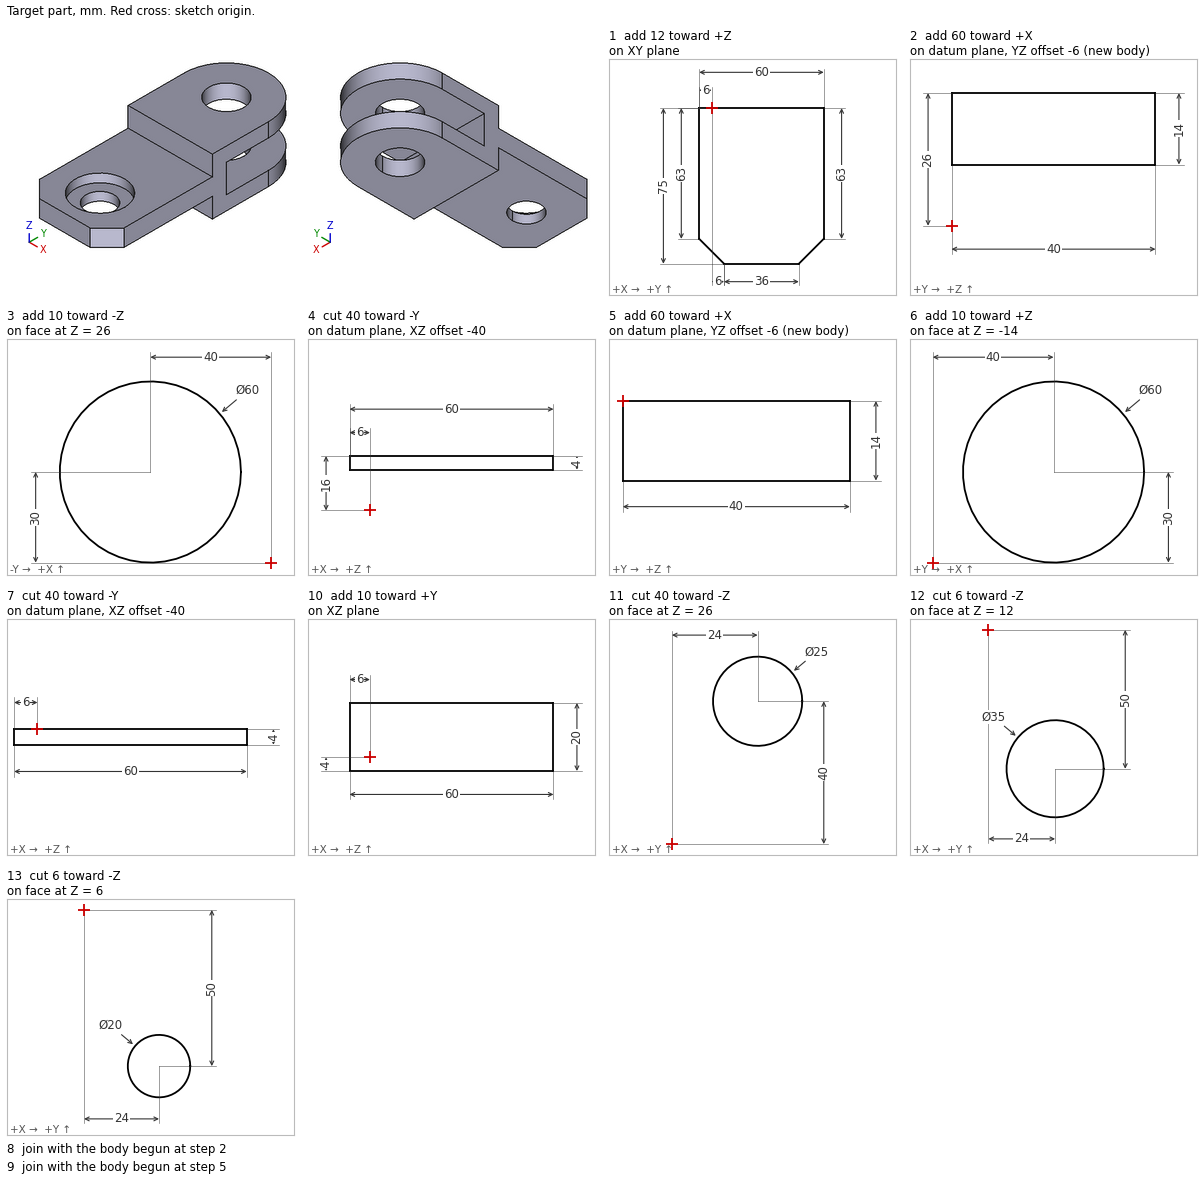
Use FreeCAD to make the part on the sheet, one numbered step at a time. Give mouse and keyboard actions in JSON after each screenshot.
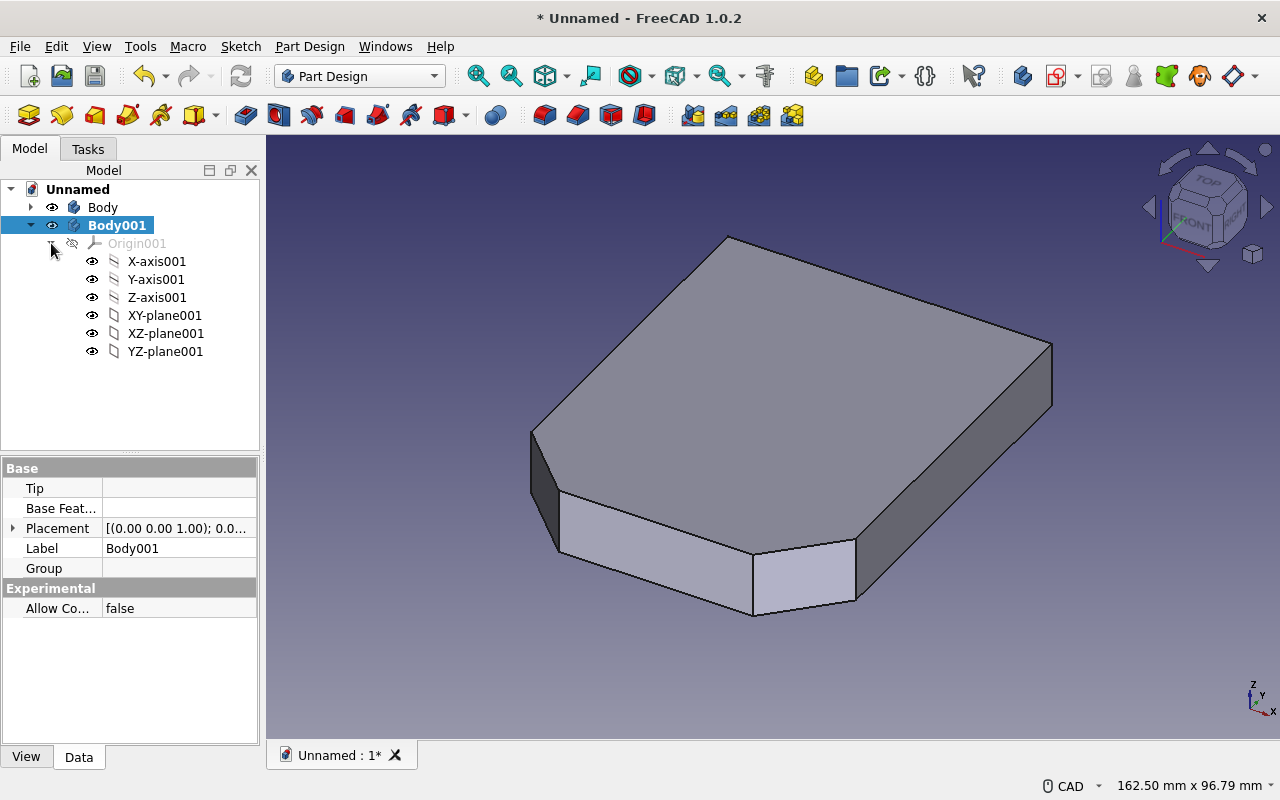
{"action": "left_click", "coordinate": [137, 351]}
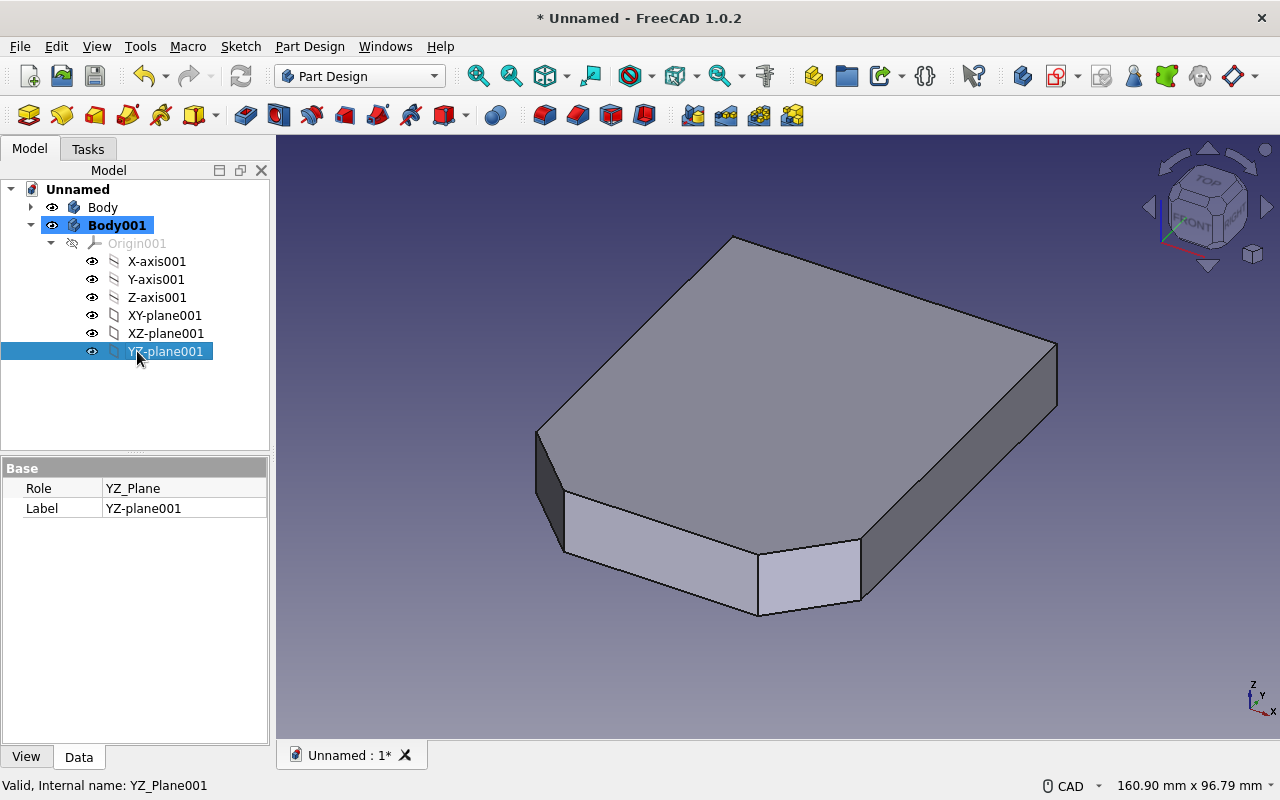
{"action": "left_click", "coordinate": [1232, 76]}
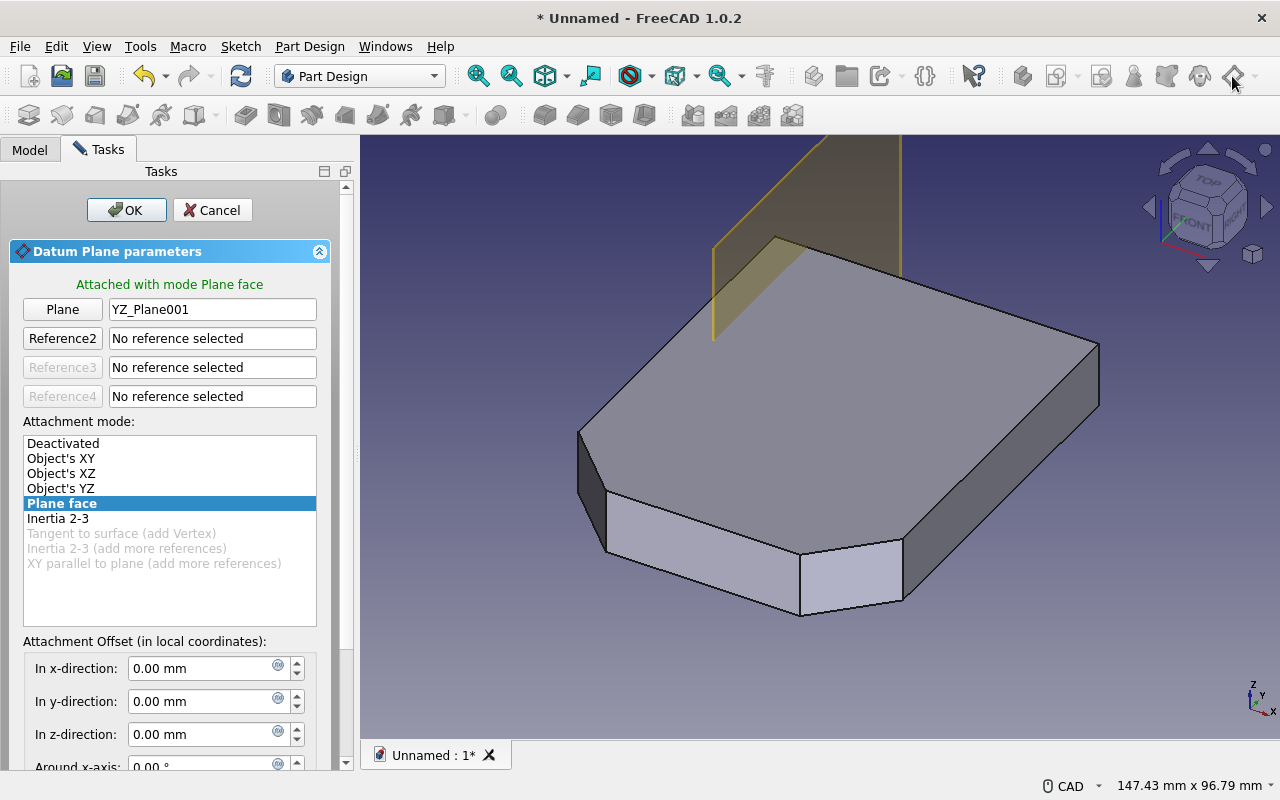
{"action": "triple_click", "coordinate": [210, 734]}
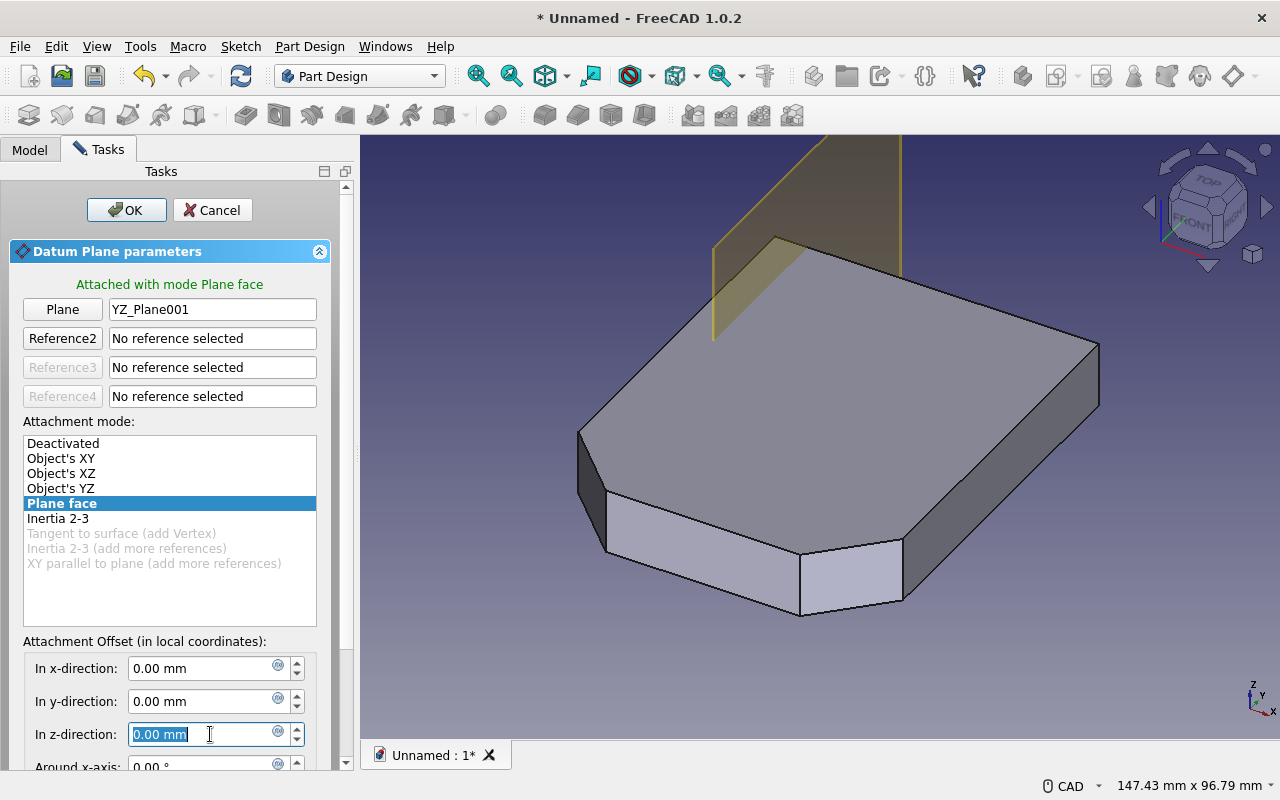
{"action": "type", "text": "-6"}
{"action": "key", "text": "Tab"}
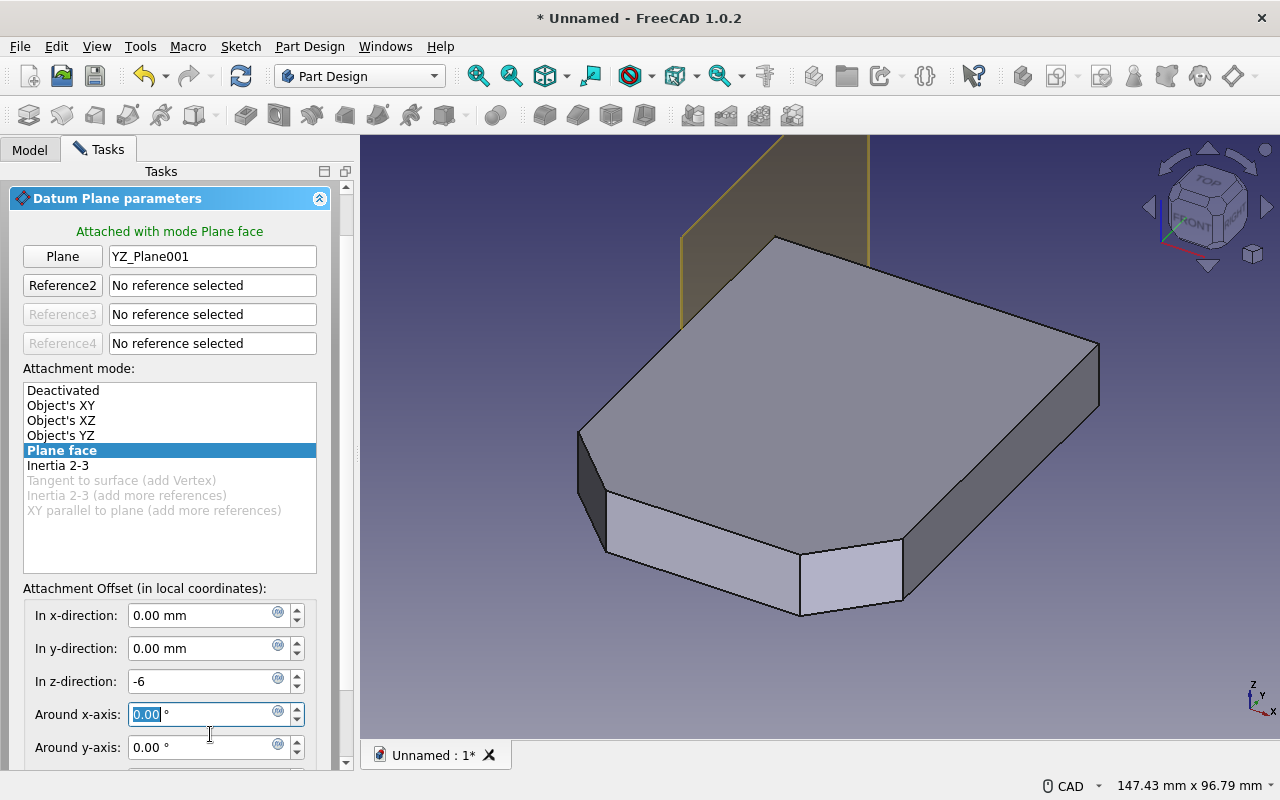
{"action": "scroll", "coordinate": [346, 476], "scroll_direction": "up", "scroll_amount": 2}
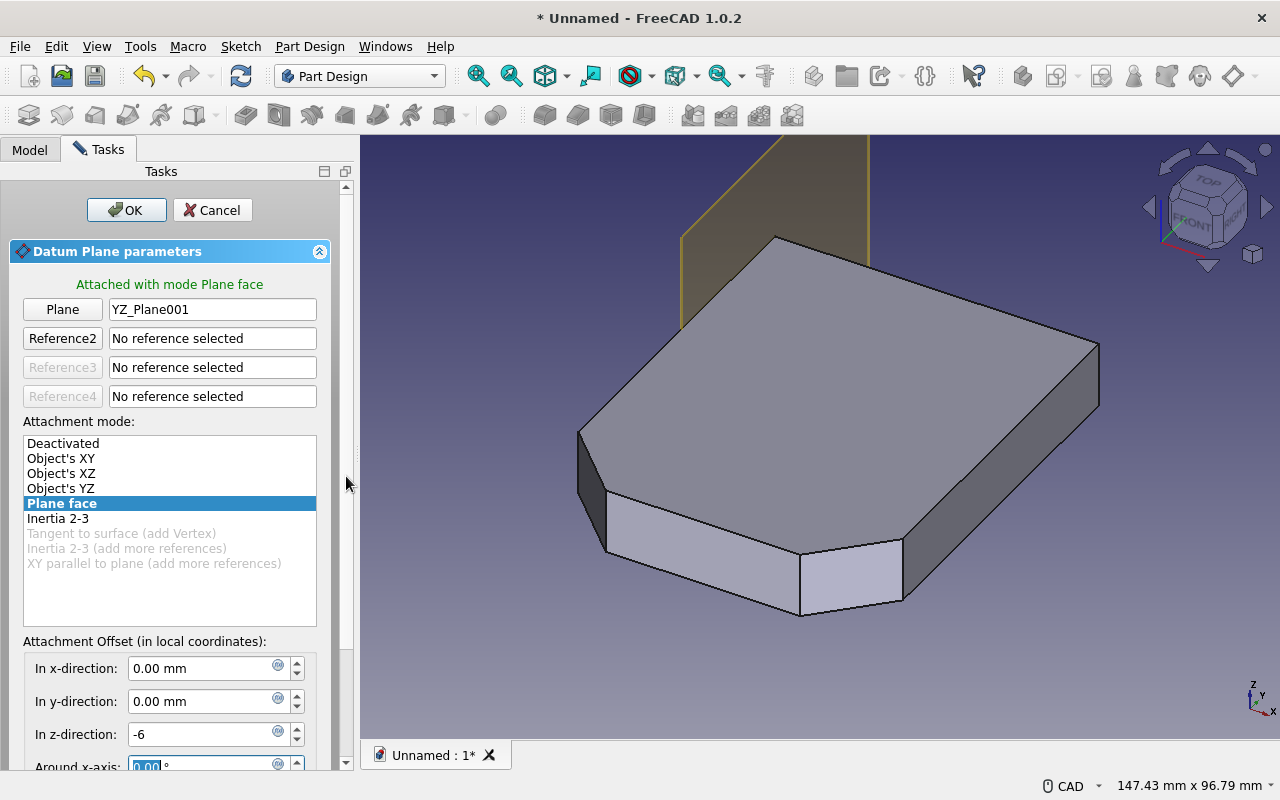
{"action": "left_click", "coordinate": [127, 210]}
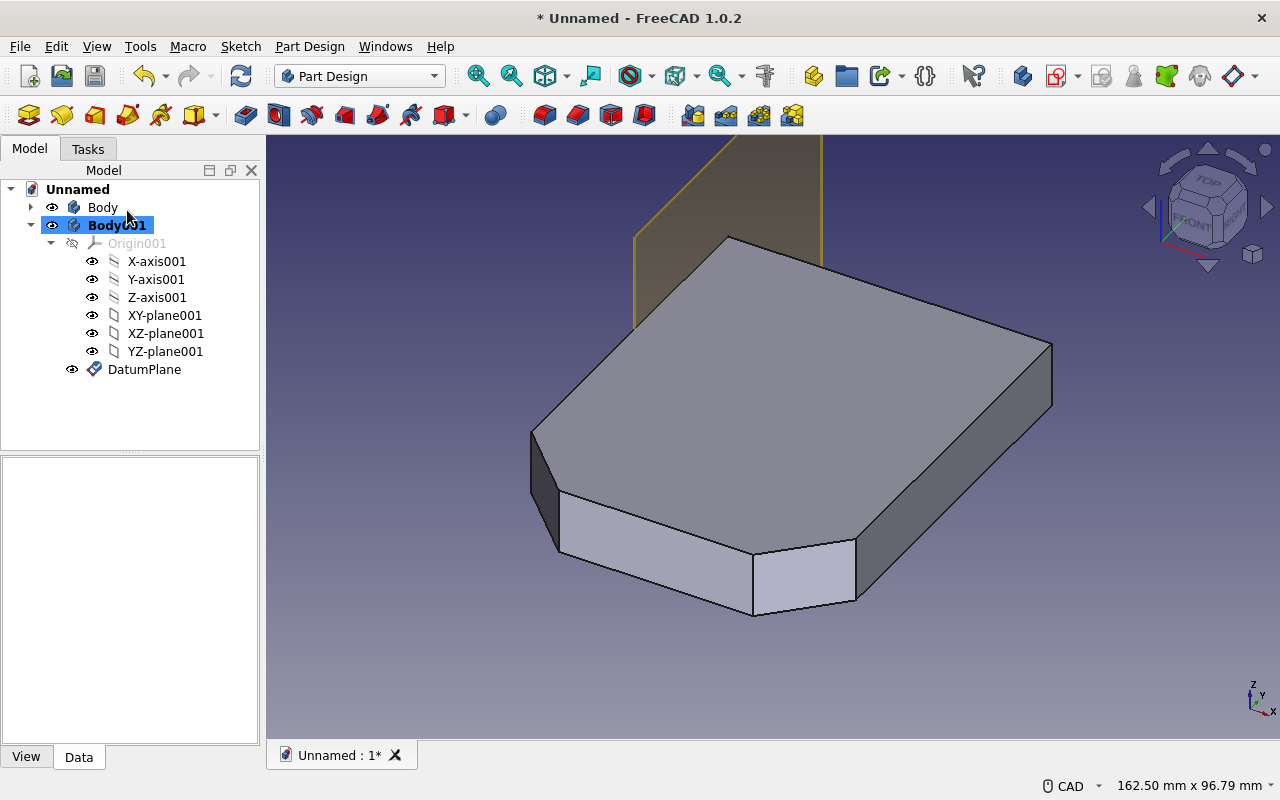
{"action": "left_click", "coordinate": [117, 369]}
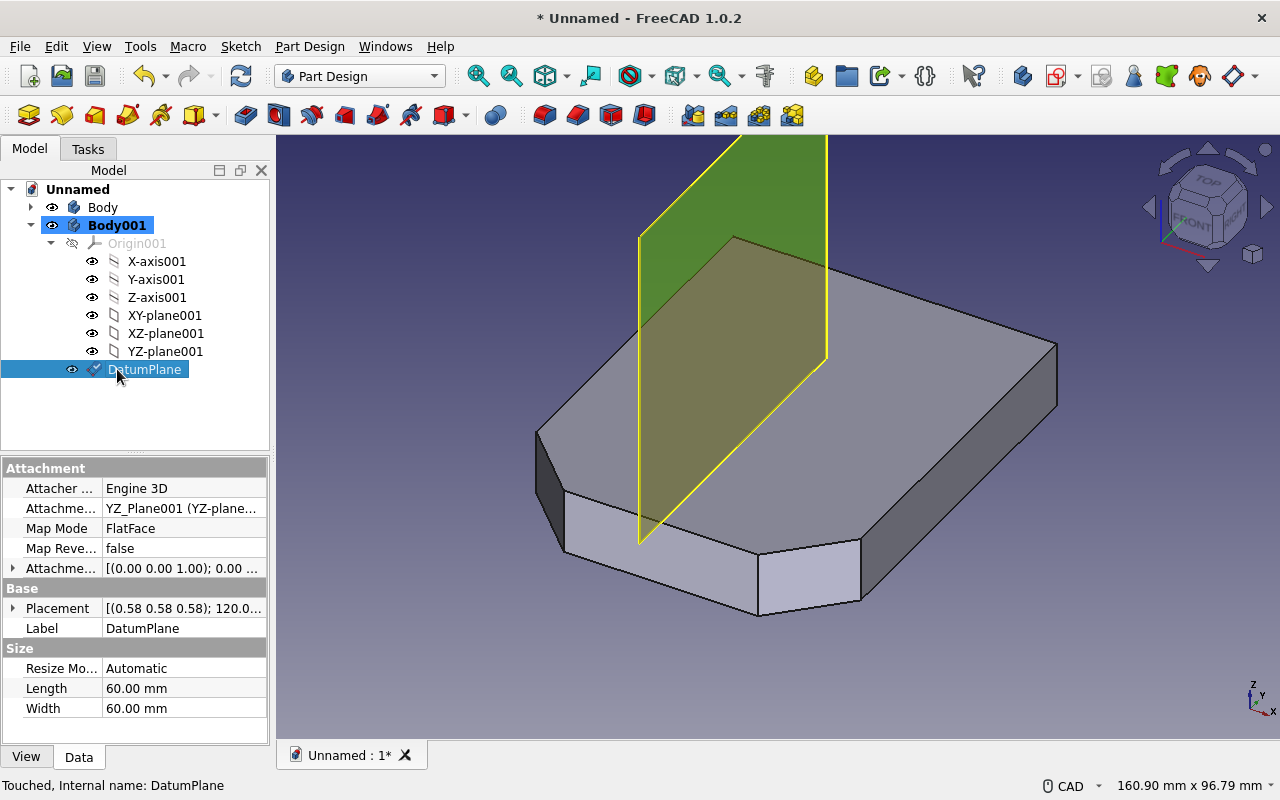
{"action": "left_click", "coordinate": [1056, 76]}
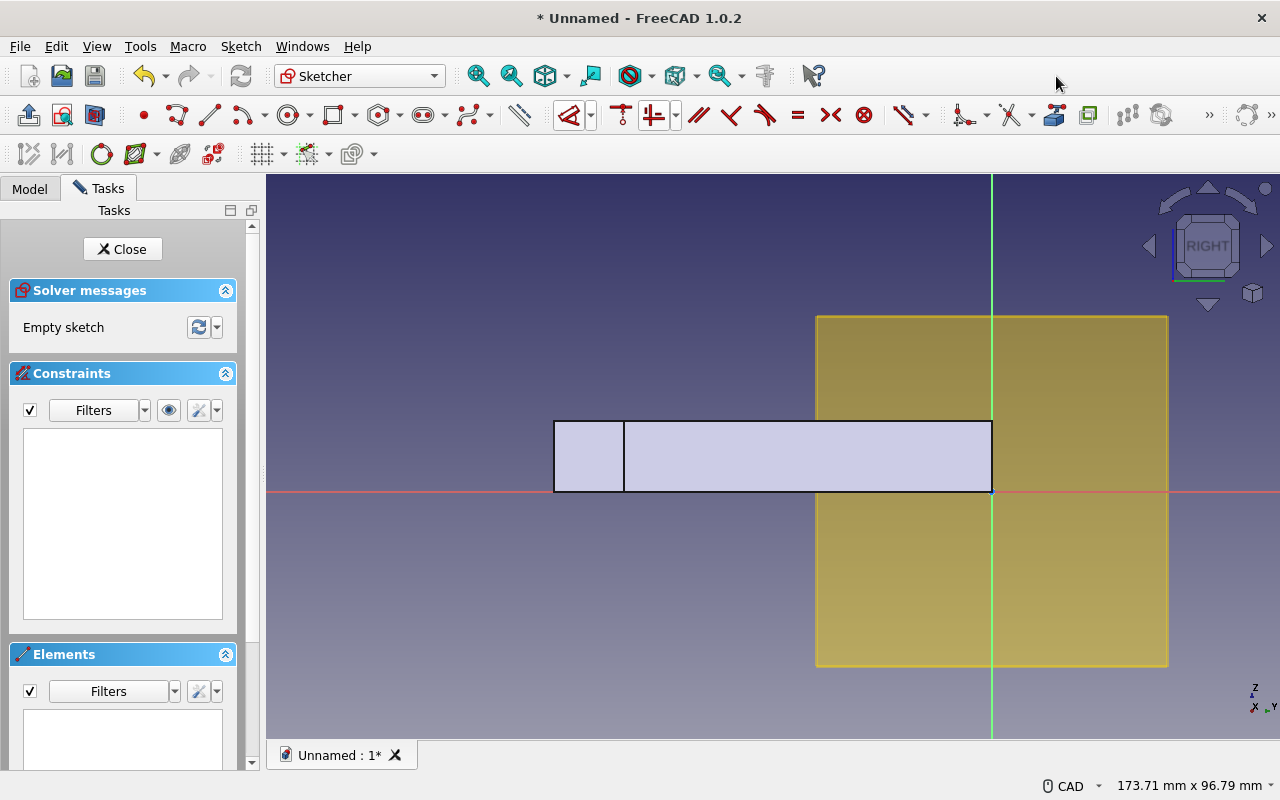
{"action": "scroll", "coordinate": [704, 456], "scroll_direction": "down", "scroll_amount": 5}